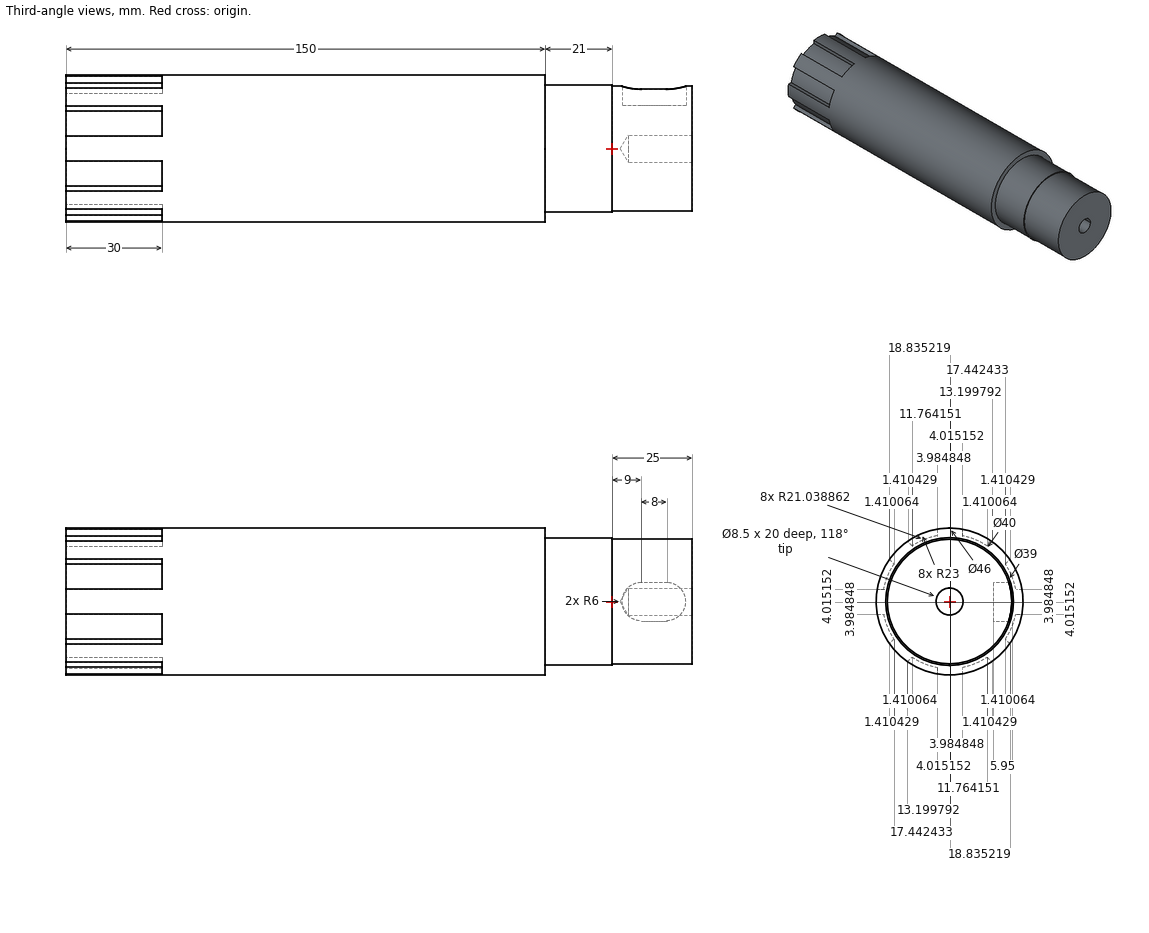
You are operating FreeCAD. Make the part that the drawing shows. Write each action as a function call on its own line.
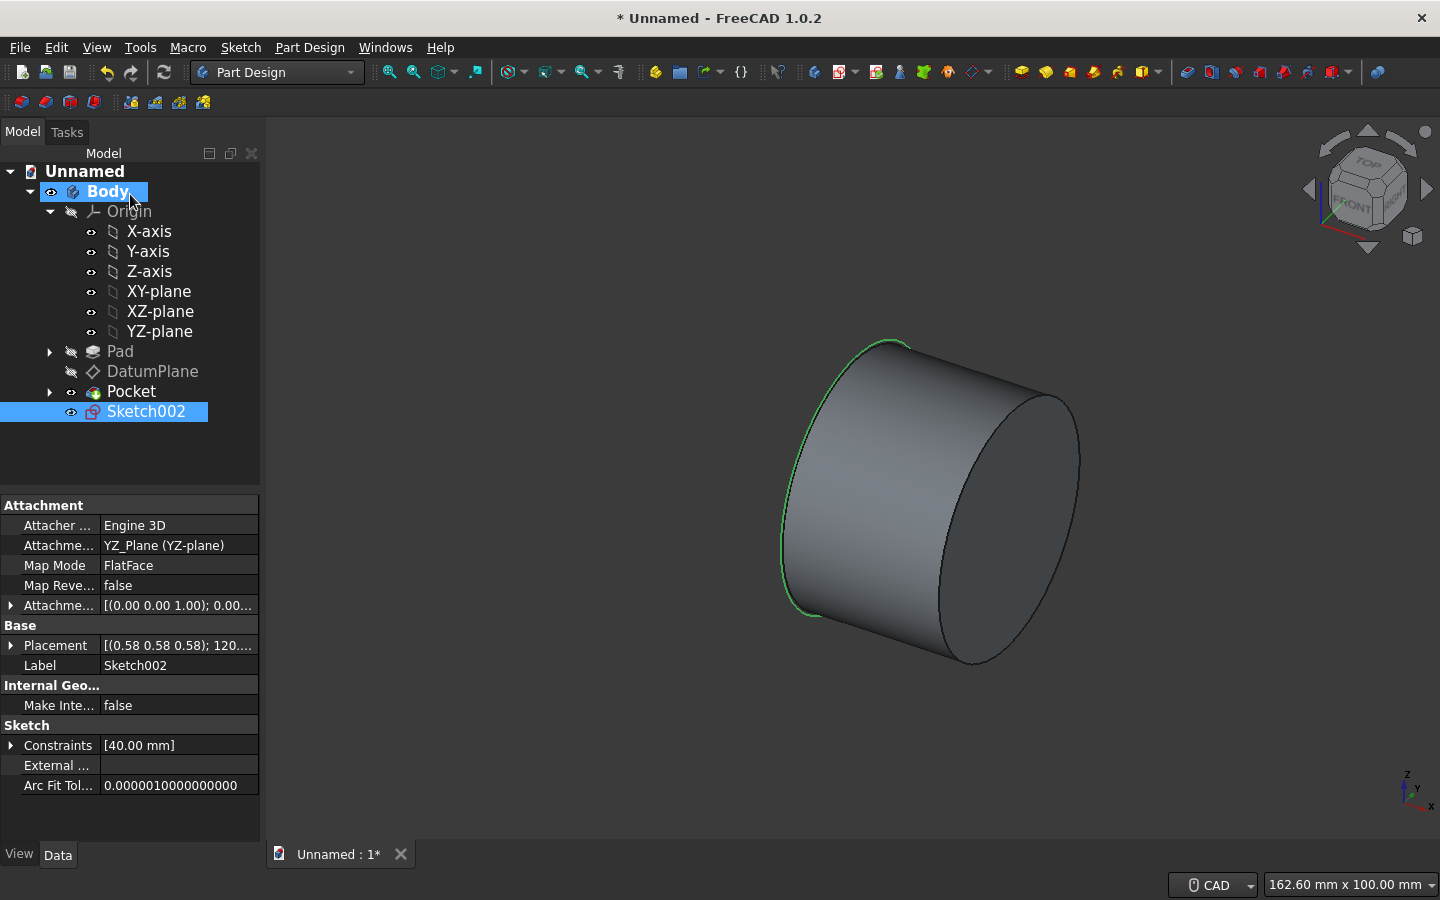
click(1022, 72)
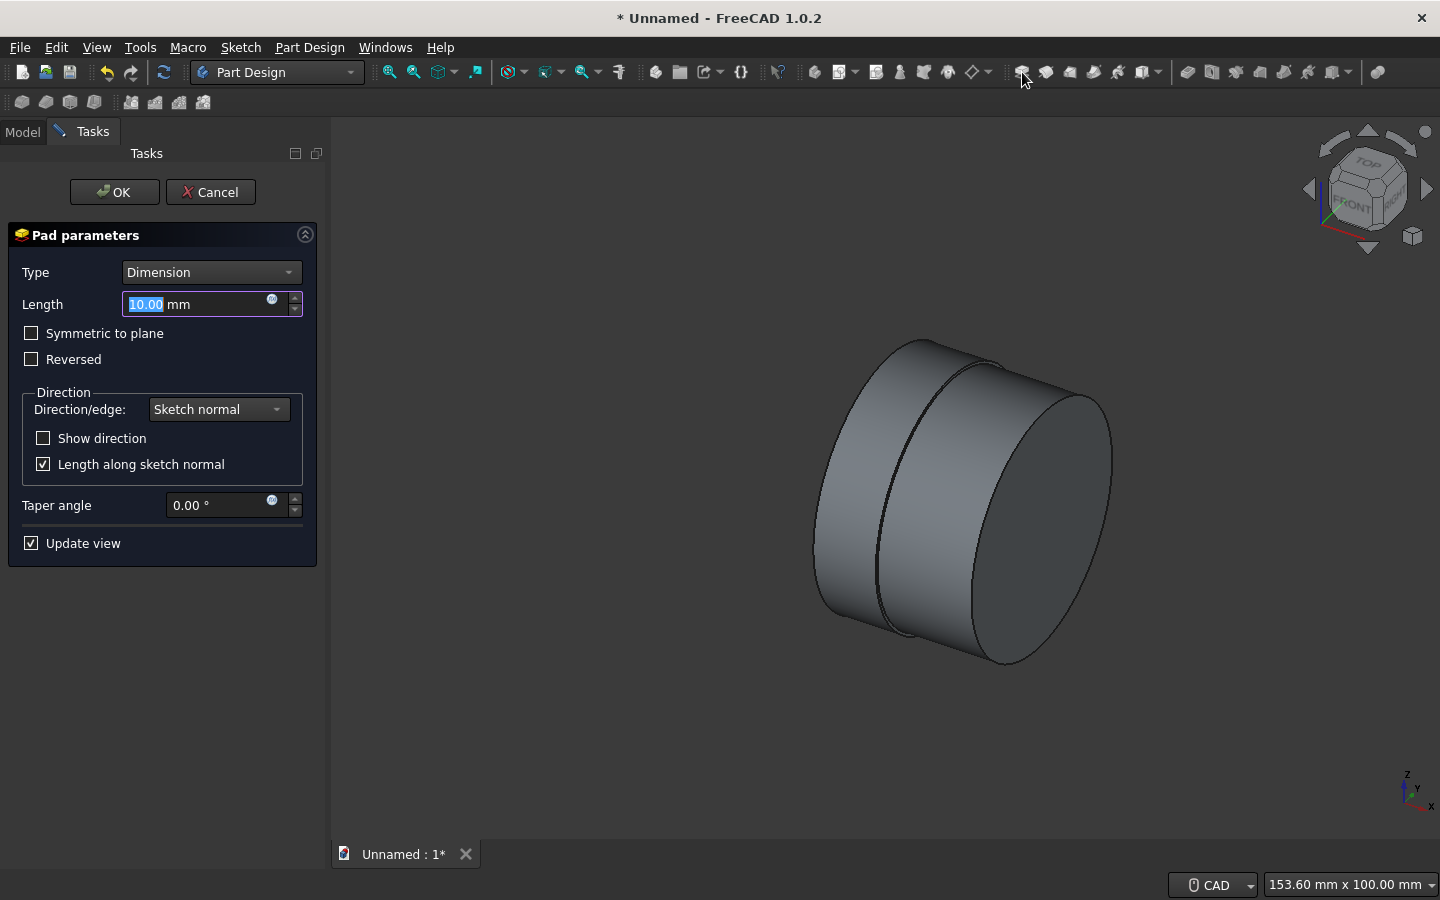
text(21)
key(Tab)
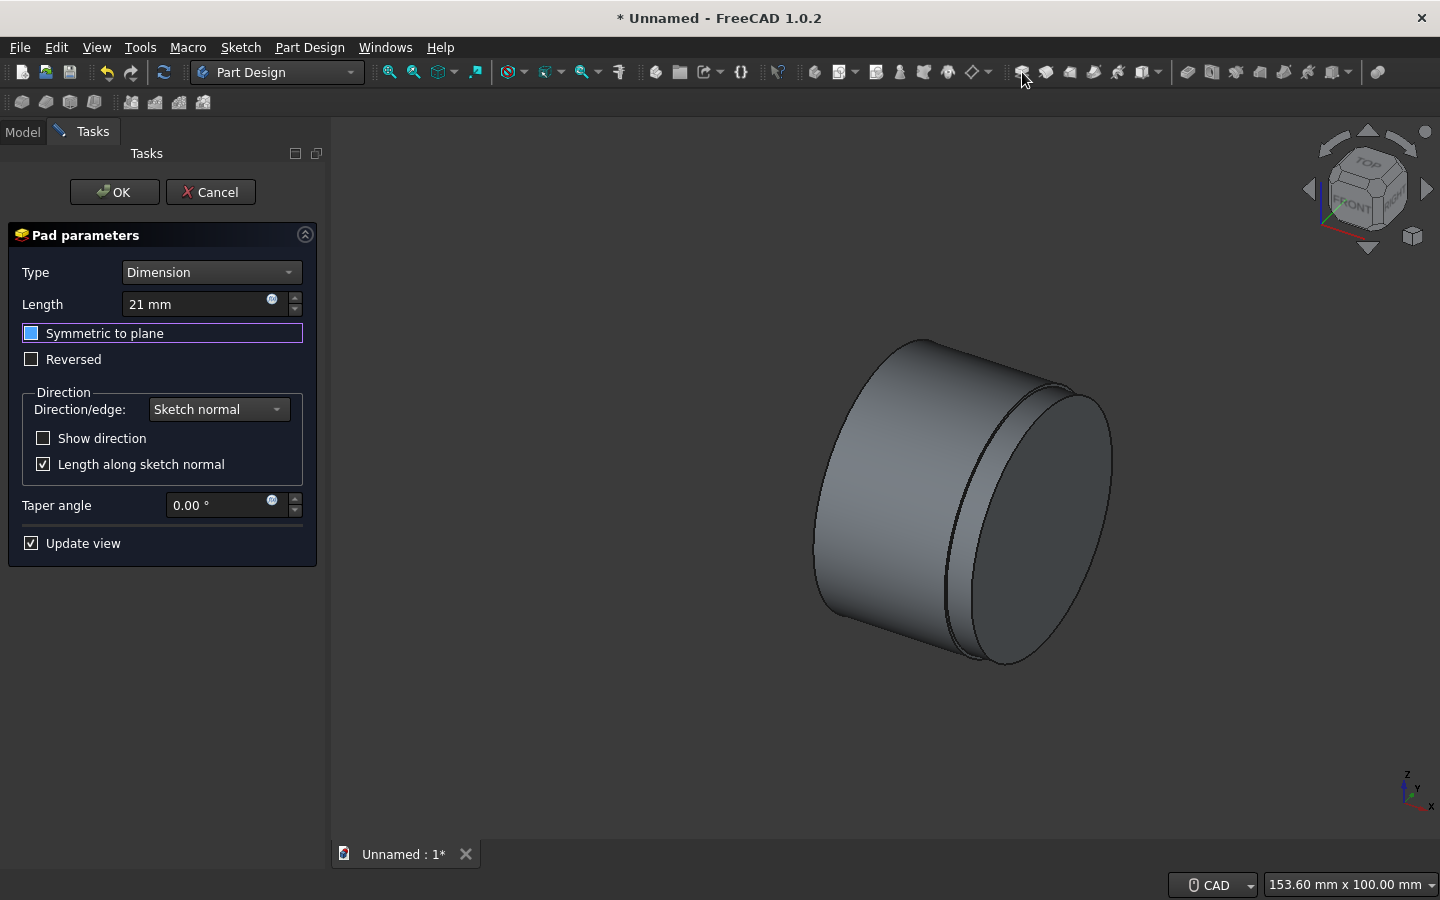
click(30, 359)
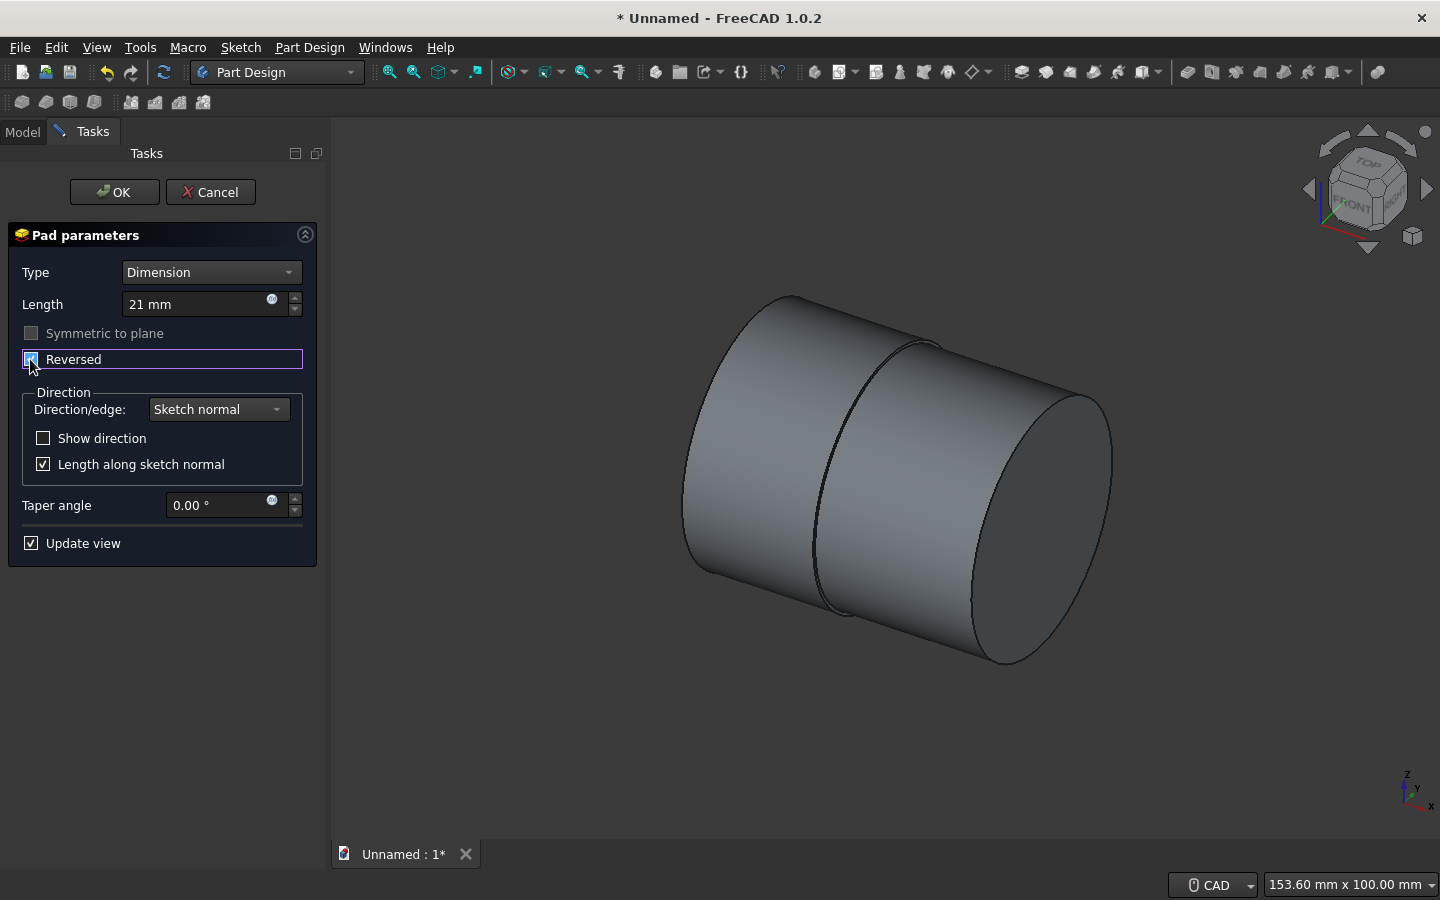
click(115, 192)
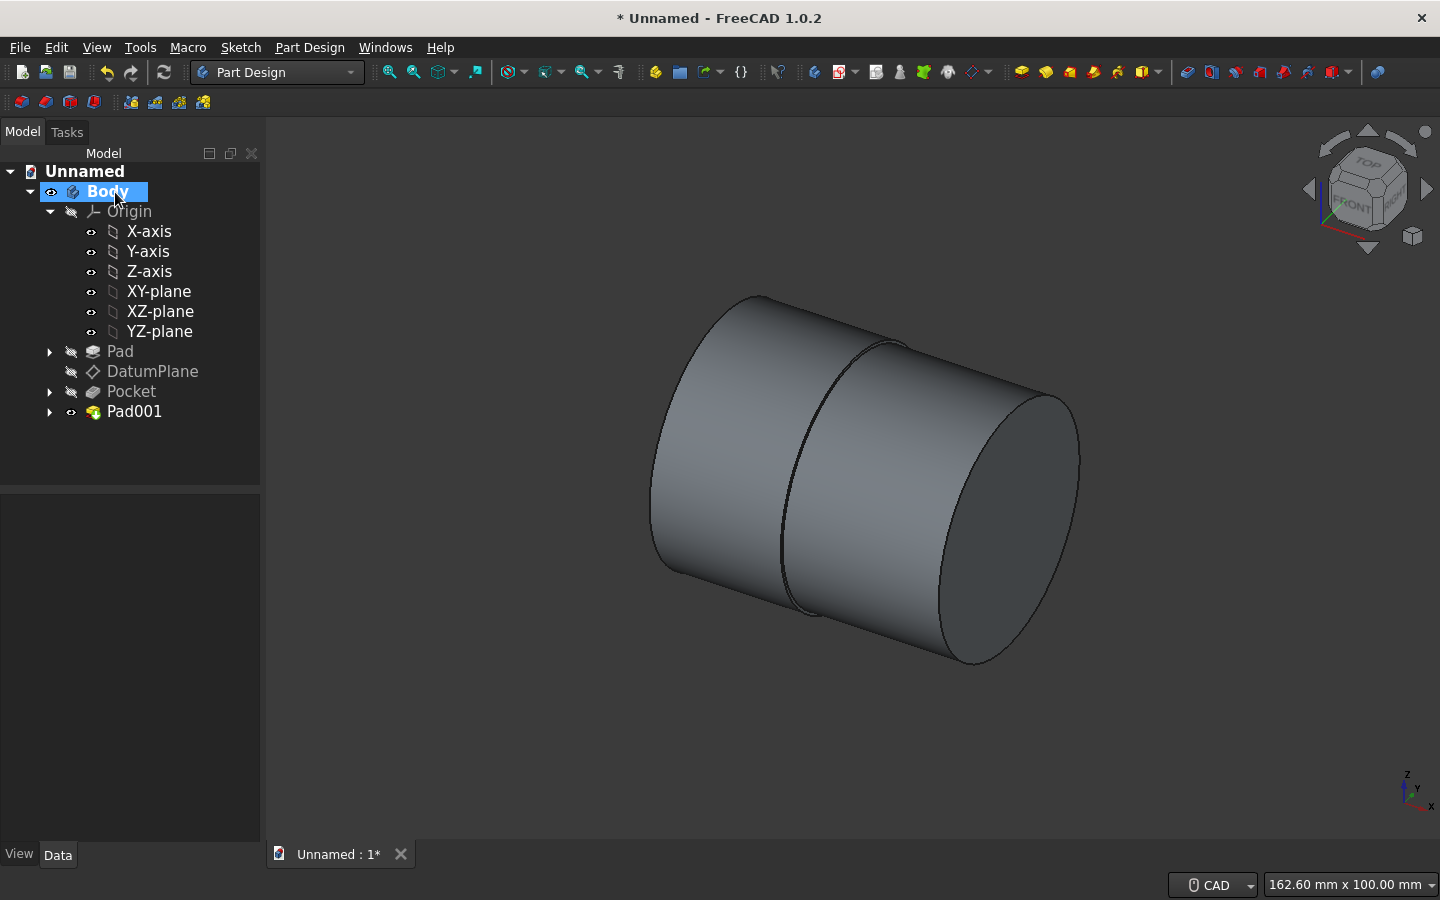
key(6)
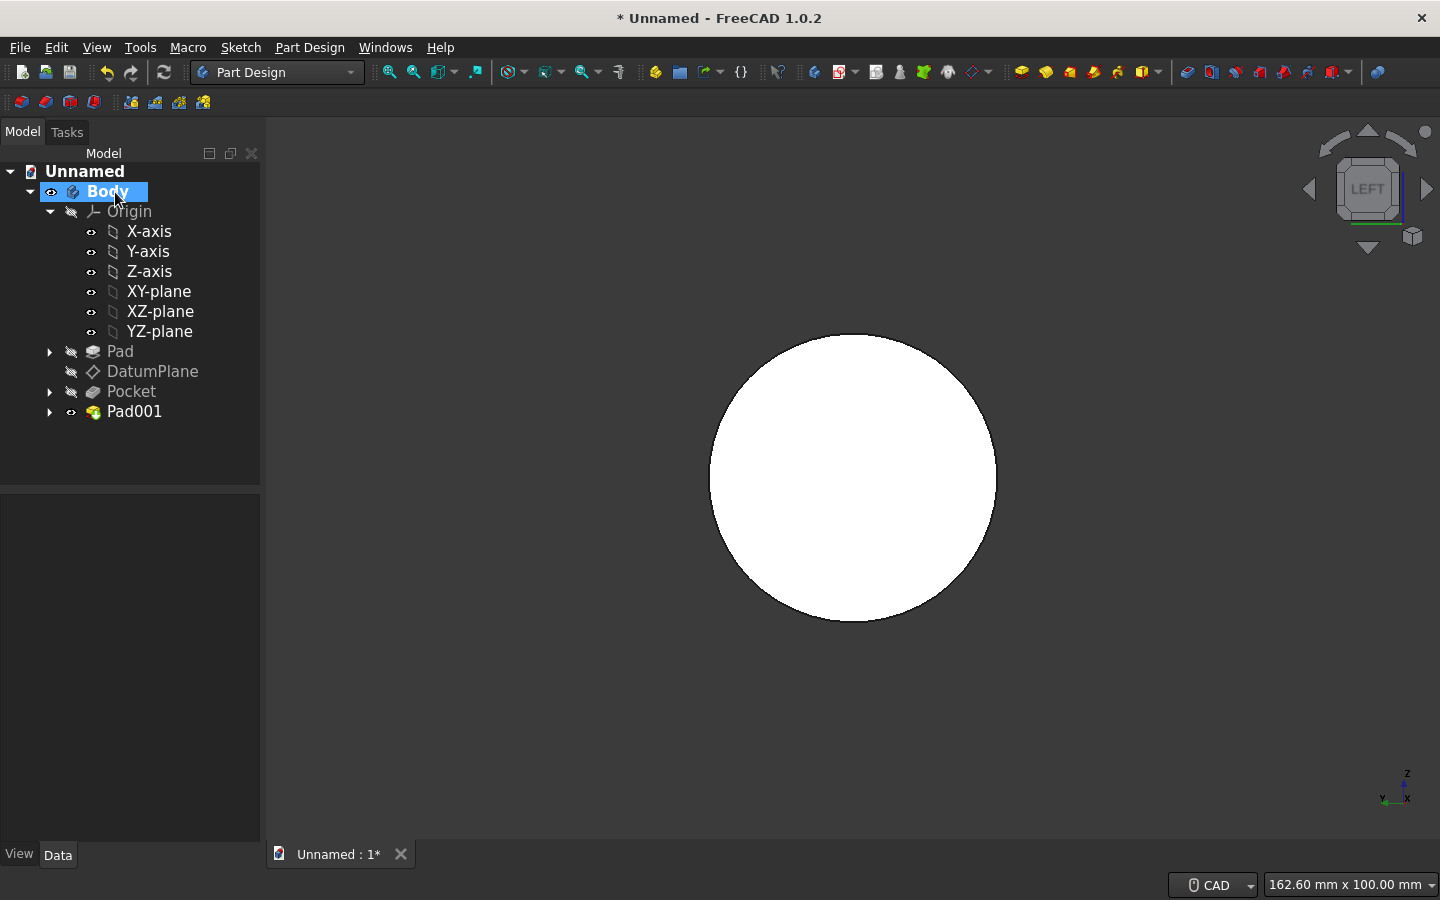
click(390, 72)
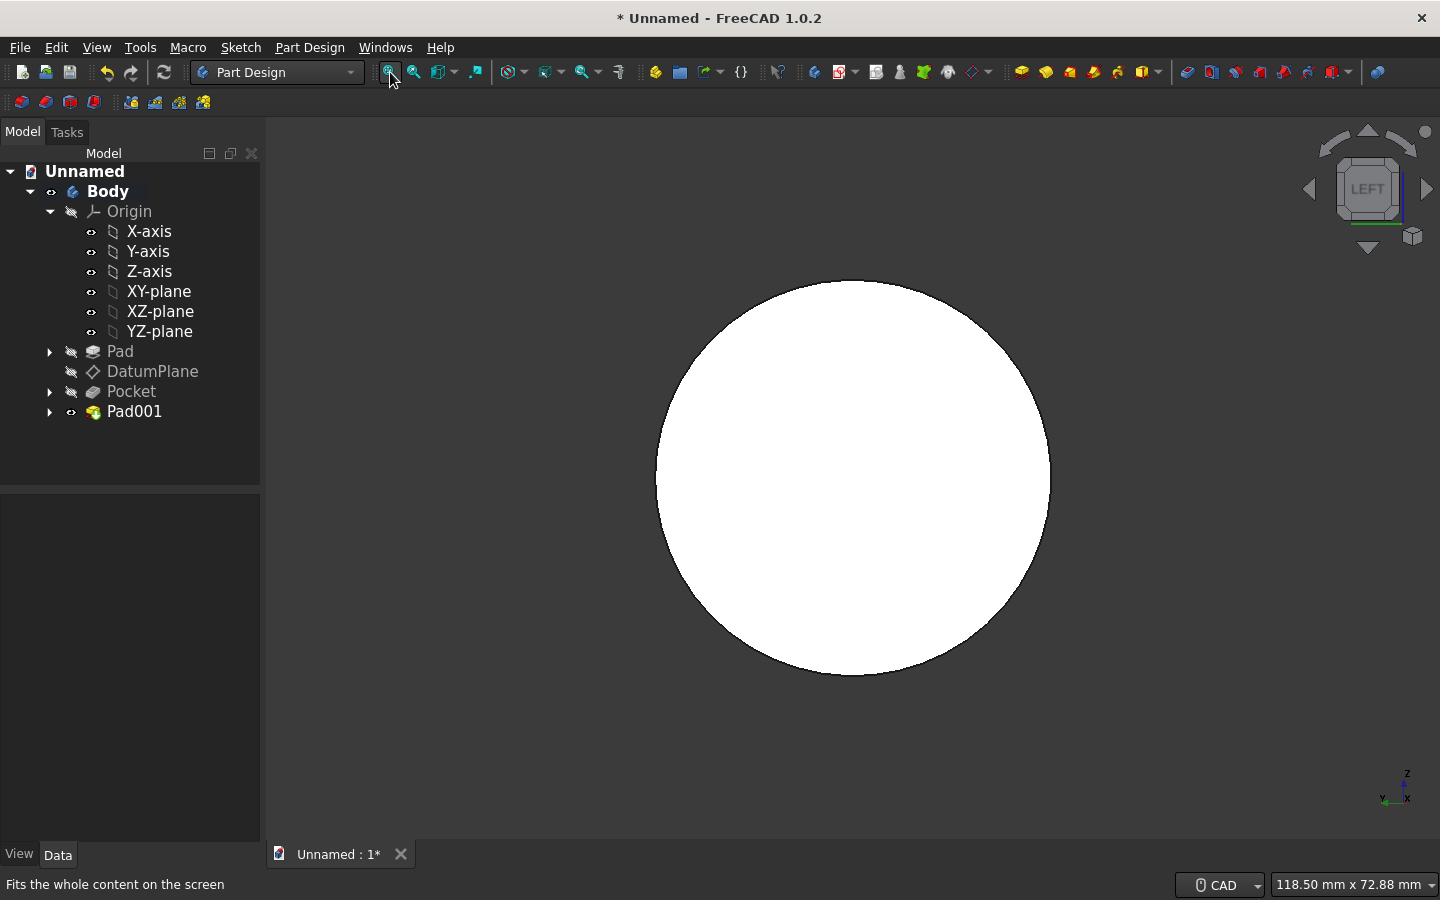
click(853, 477)